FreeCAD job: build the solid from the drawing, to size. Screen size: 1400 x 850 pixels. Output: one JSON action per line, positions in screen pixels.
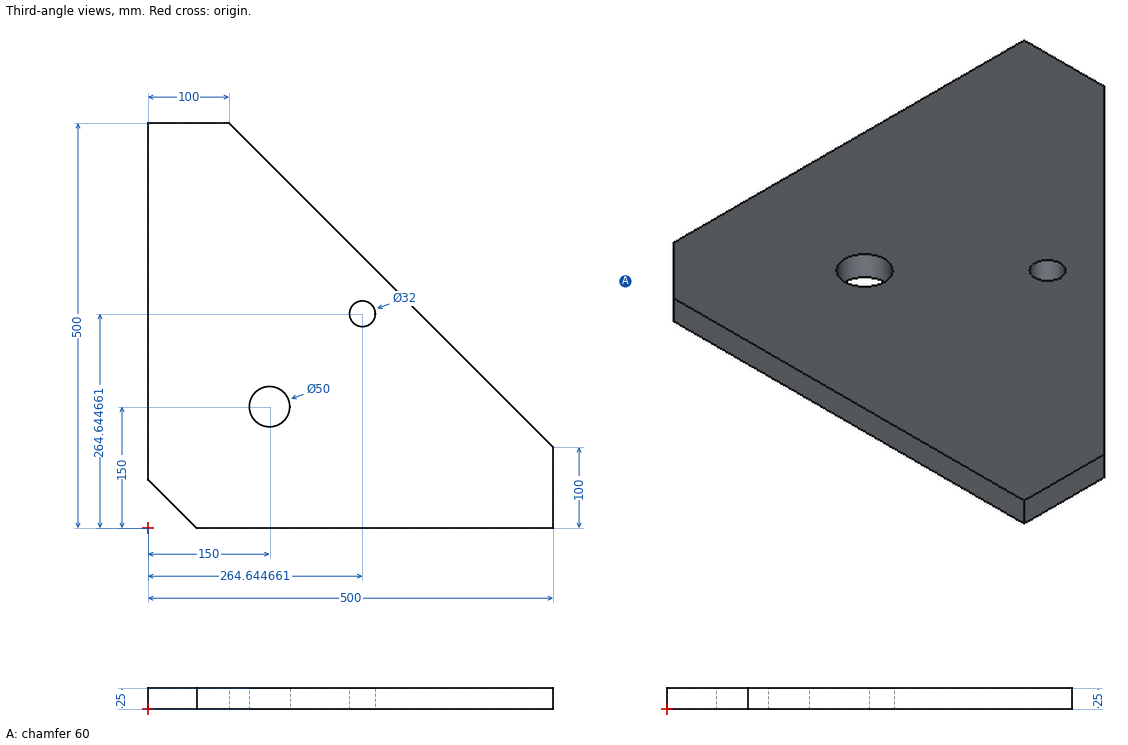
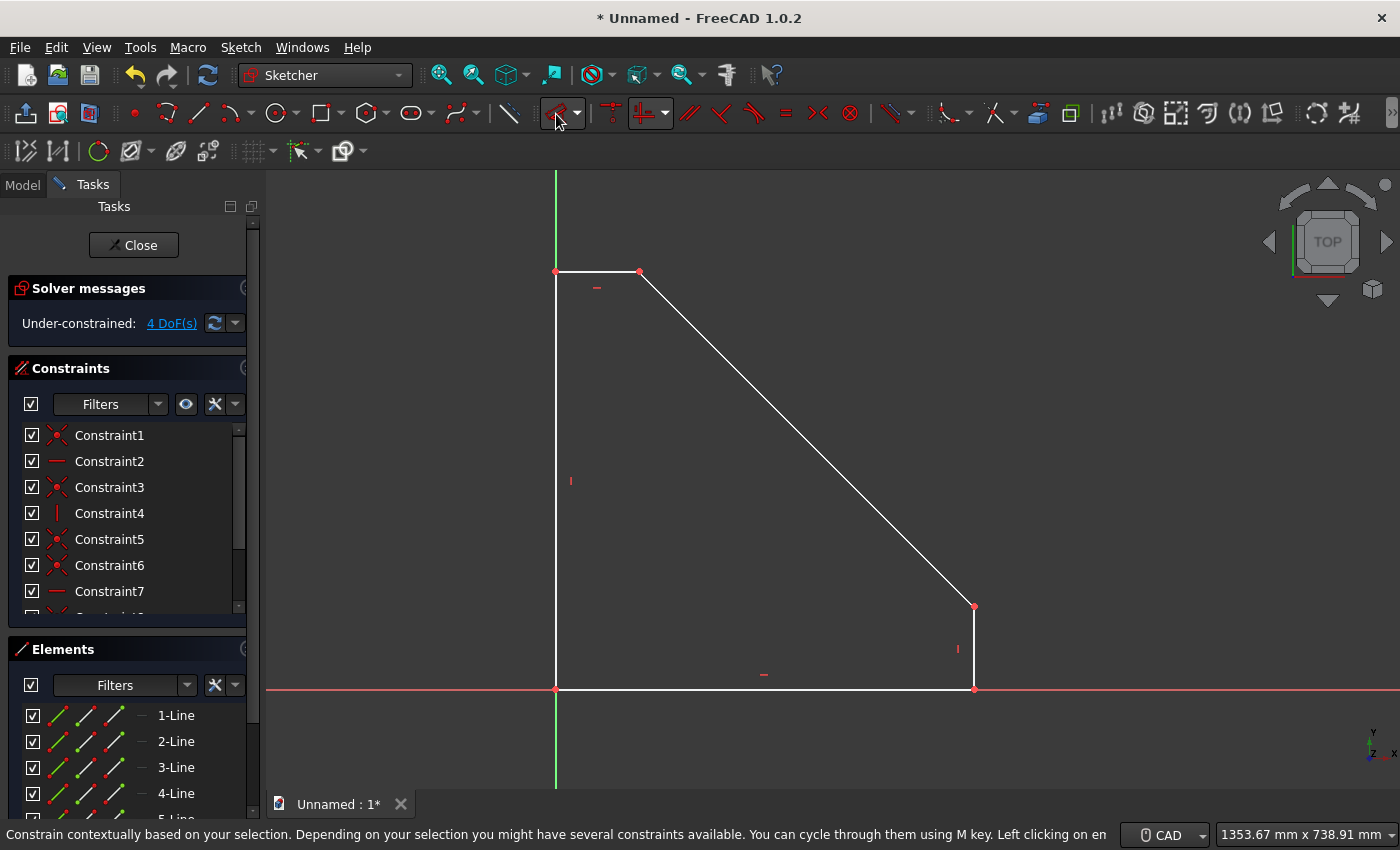
{"action": "left_click", "coordinate": [681, 690]}
{"action": "left_click", "coordinate": [765, 724]}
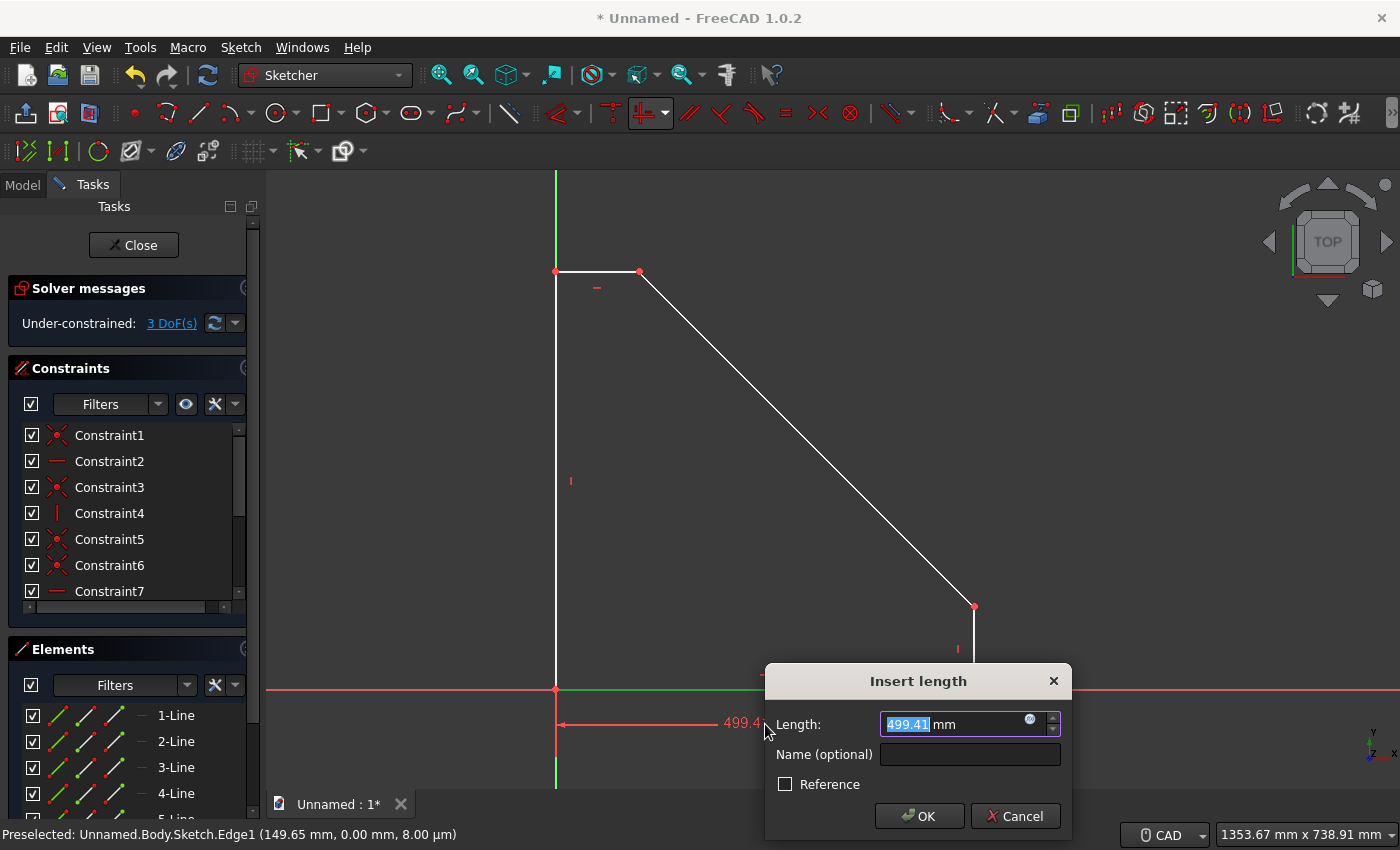
{"action": "type", "text": "500"}
{"action": "key", "text": "Return"}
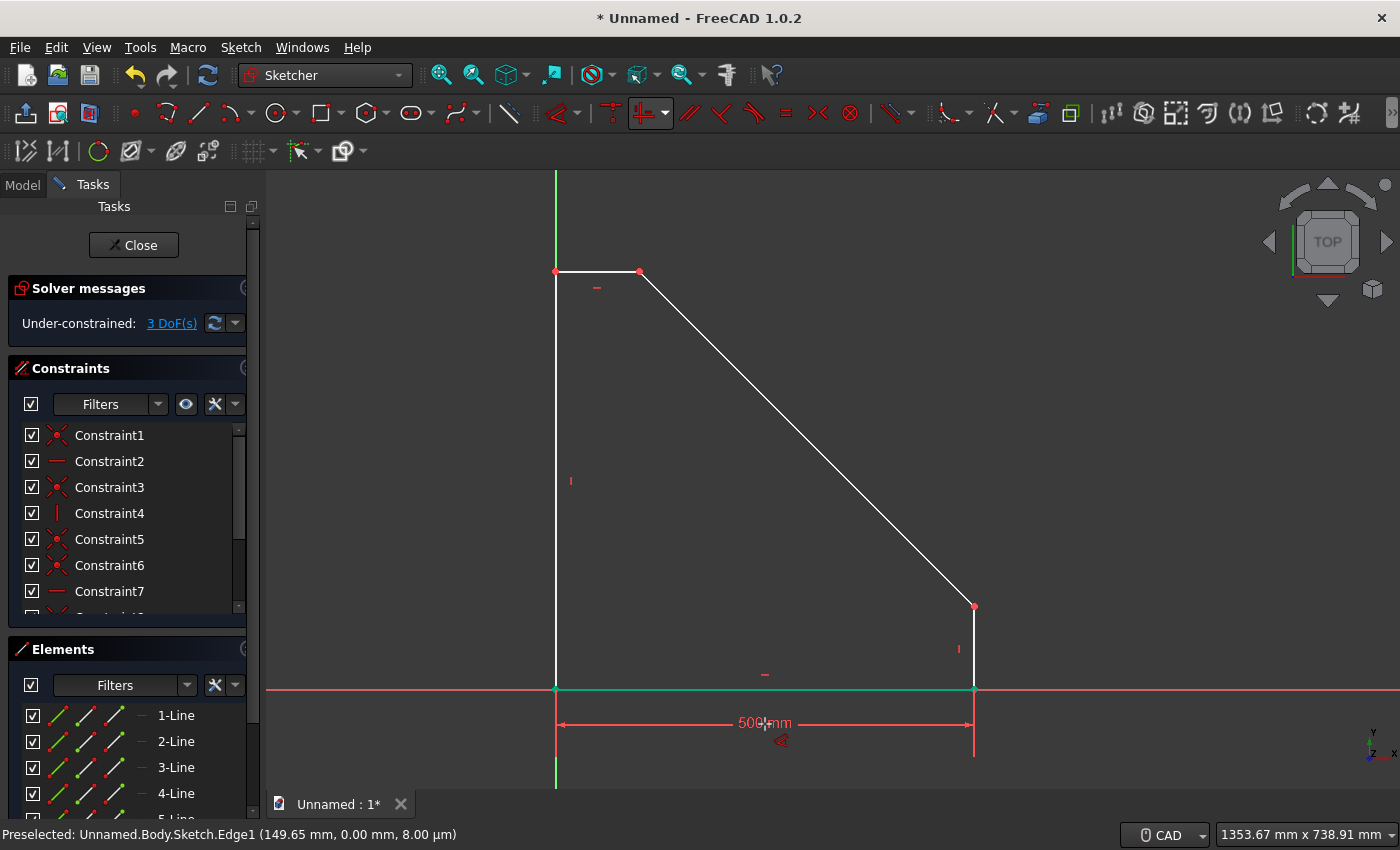
{"action": "left_click", "coordinate": [974, 665]}
{"action": "left_click", "coordinate": [1008, 648]}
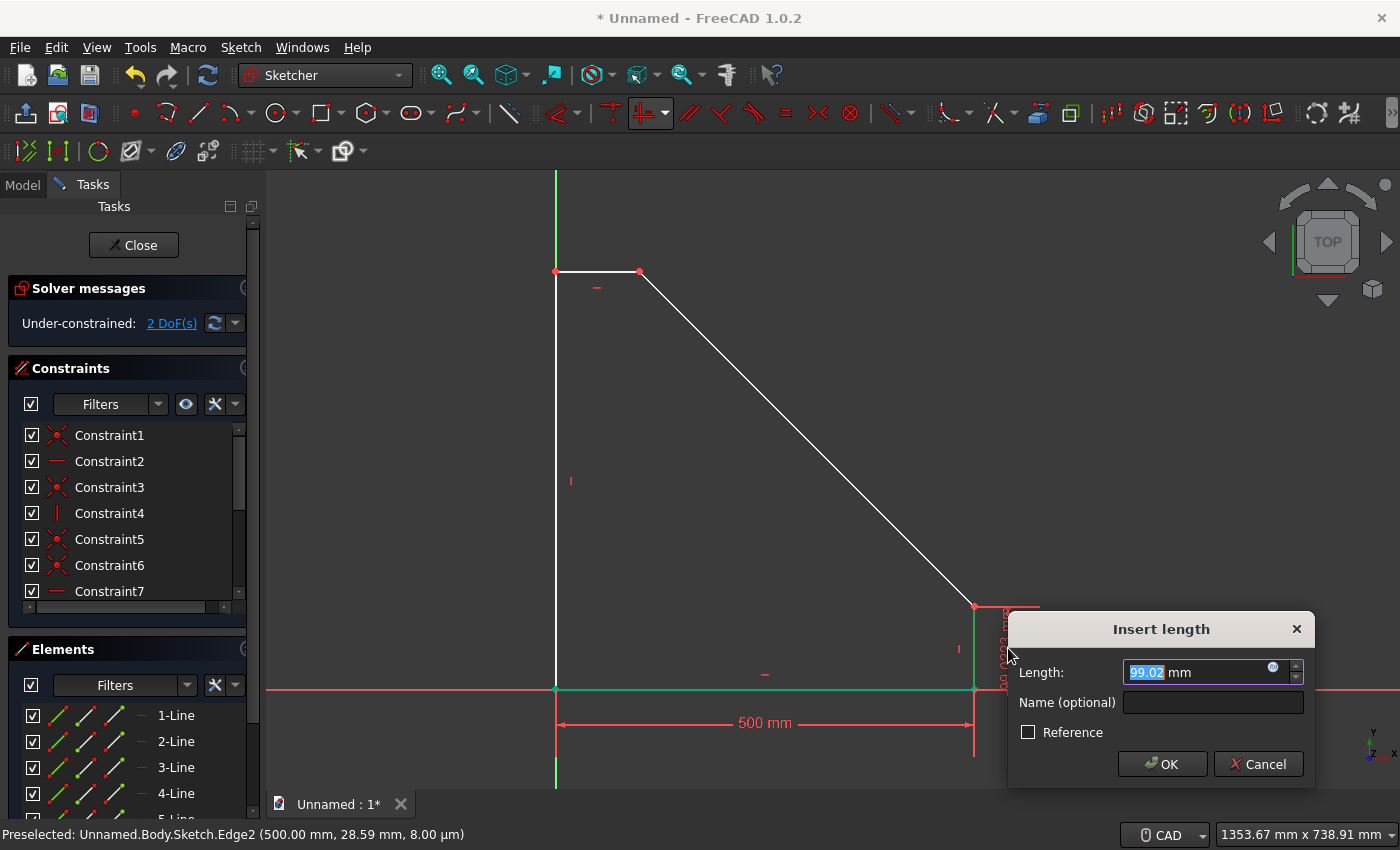
{"action": "type", "text": "100"}
{"action": "key", "text": "Return"}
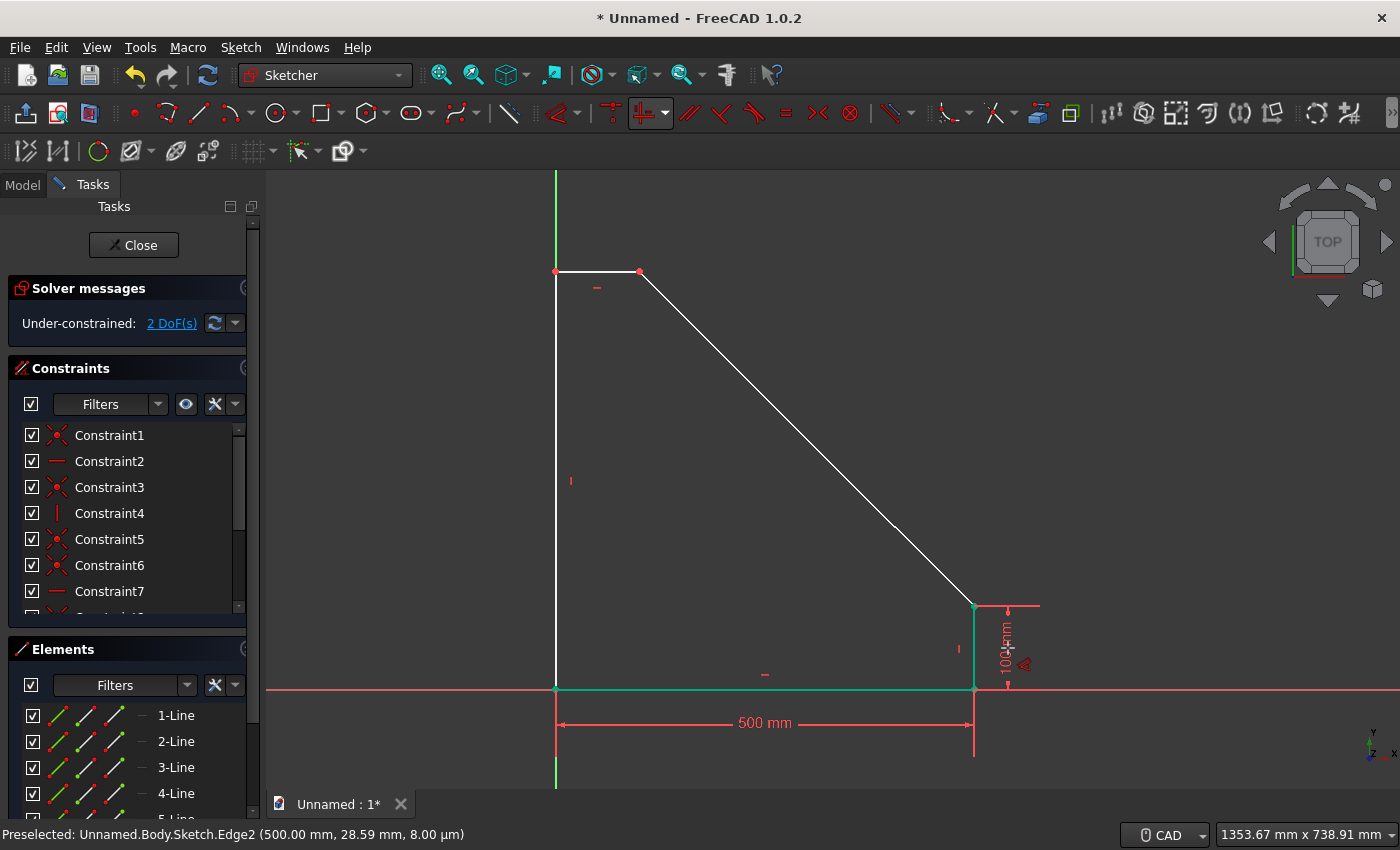
{"action": "left_click", "coordinate": [614, 272]}
{"action": "left_click", "coordinate": [597, 238]}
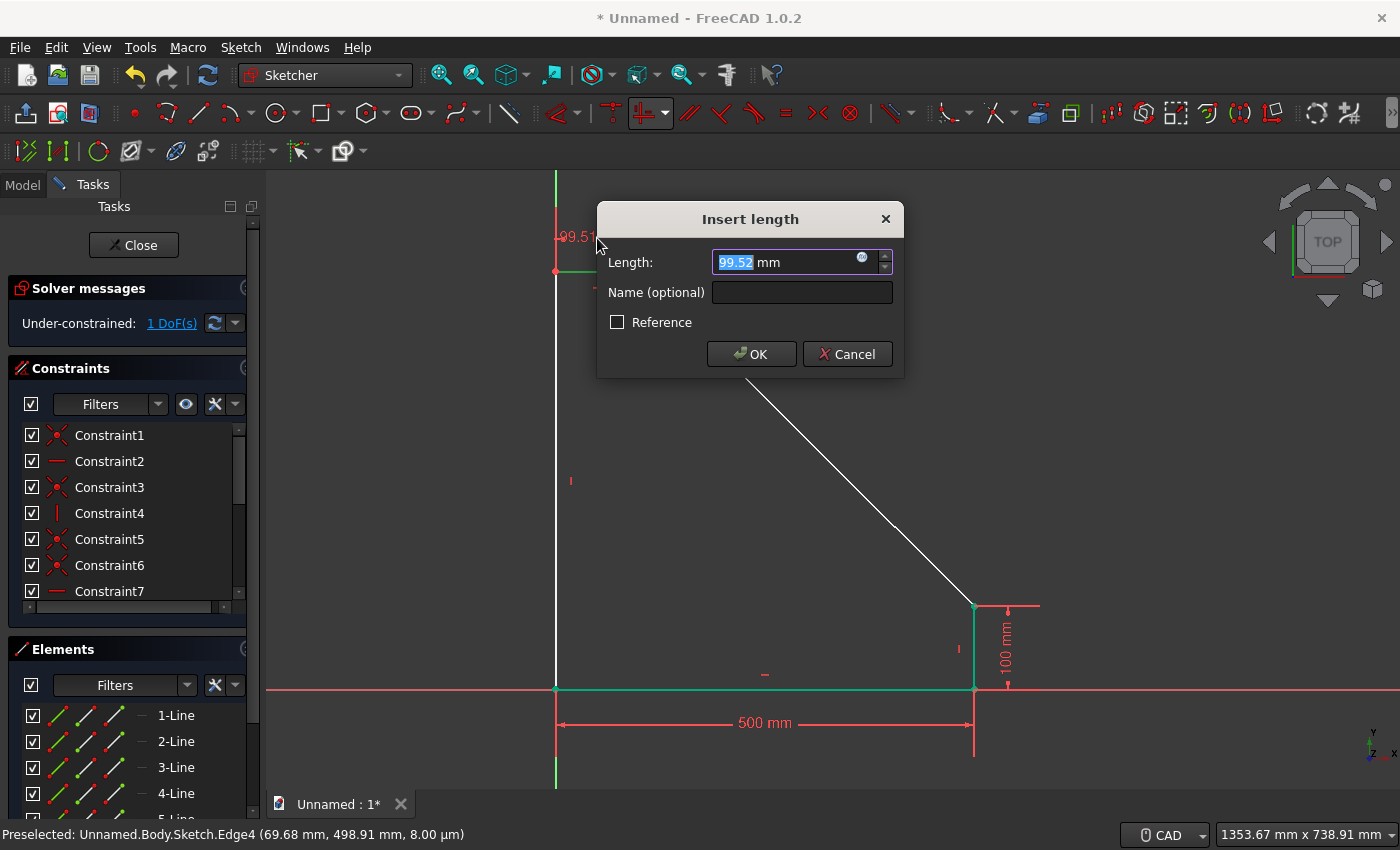
{"action": "type", "text": "100"}
{"action": "key", "text": "Return"}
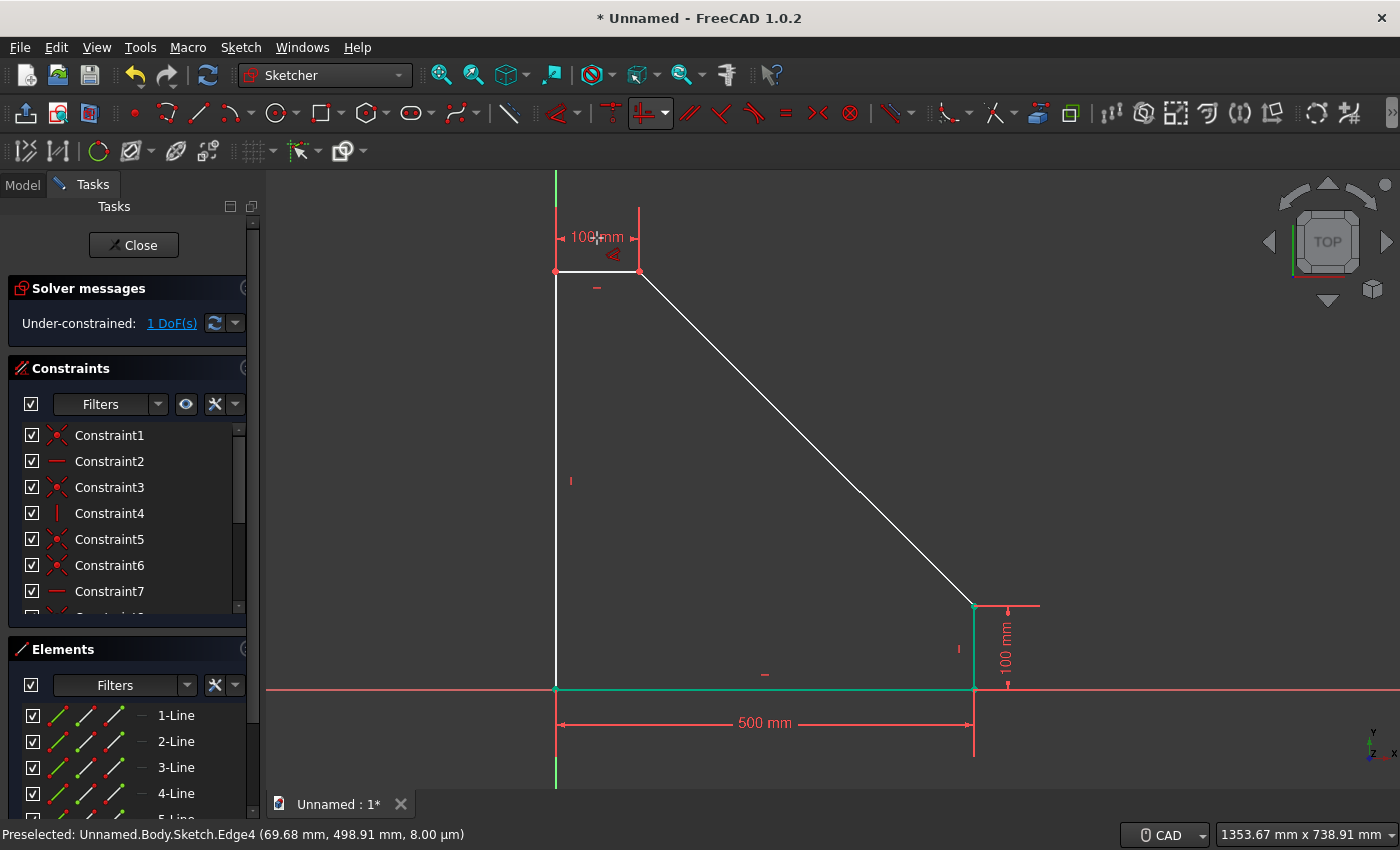
{"action": "left_click", "coordinate": [556, 397]}
{"action": "left_click", "coordinate": [522, 481]}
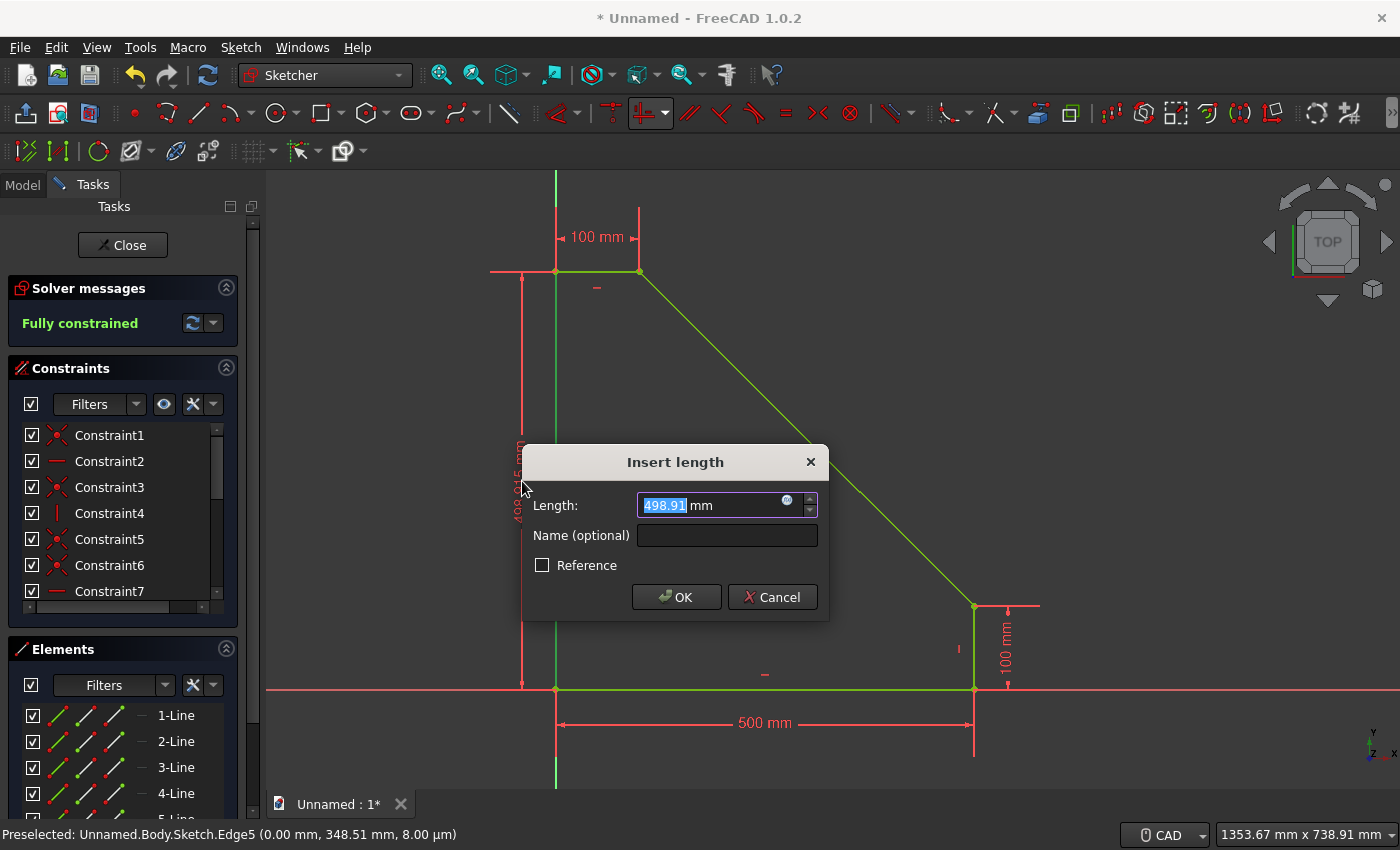
{"action": "type", "text": "500"}
{"action": "key", "text": "Return"}
{"action": "key", "text": "Escape"}